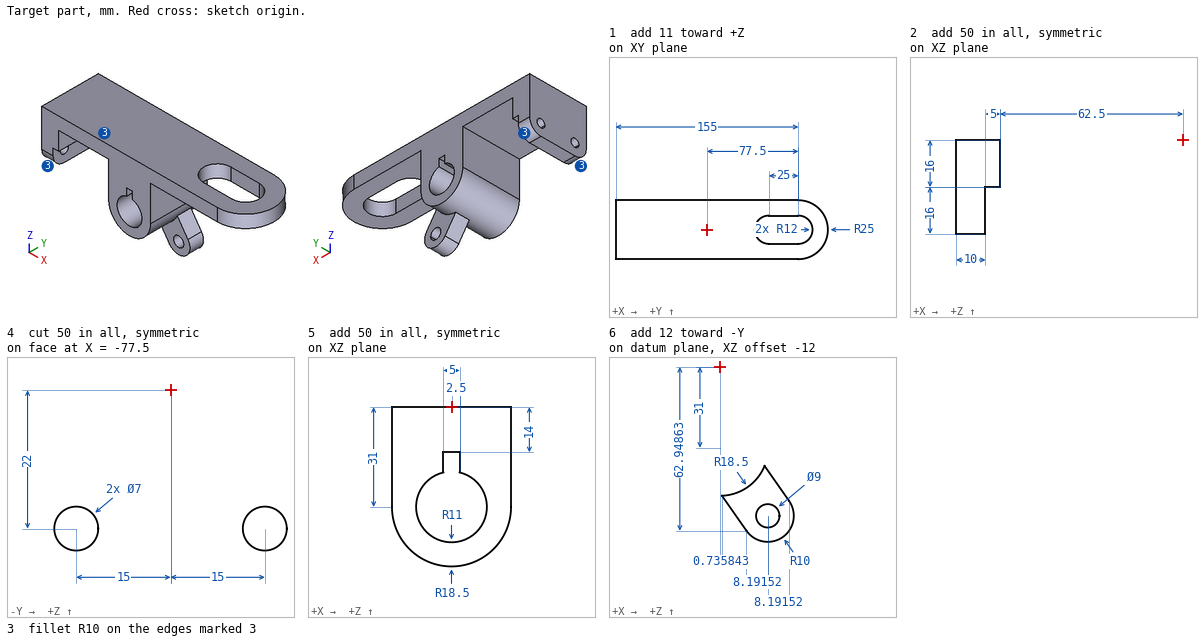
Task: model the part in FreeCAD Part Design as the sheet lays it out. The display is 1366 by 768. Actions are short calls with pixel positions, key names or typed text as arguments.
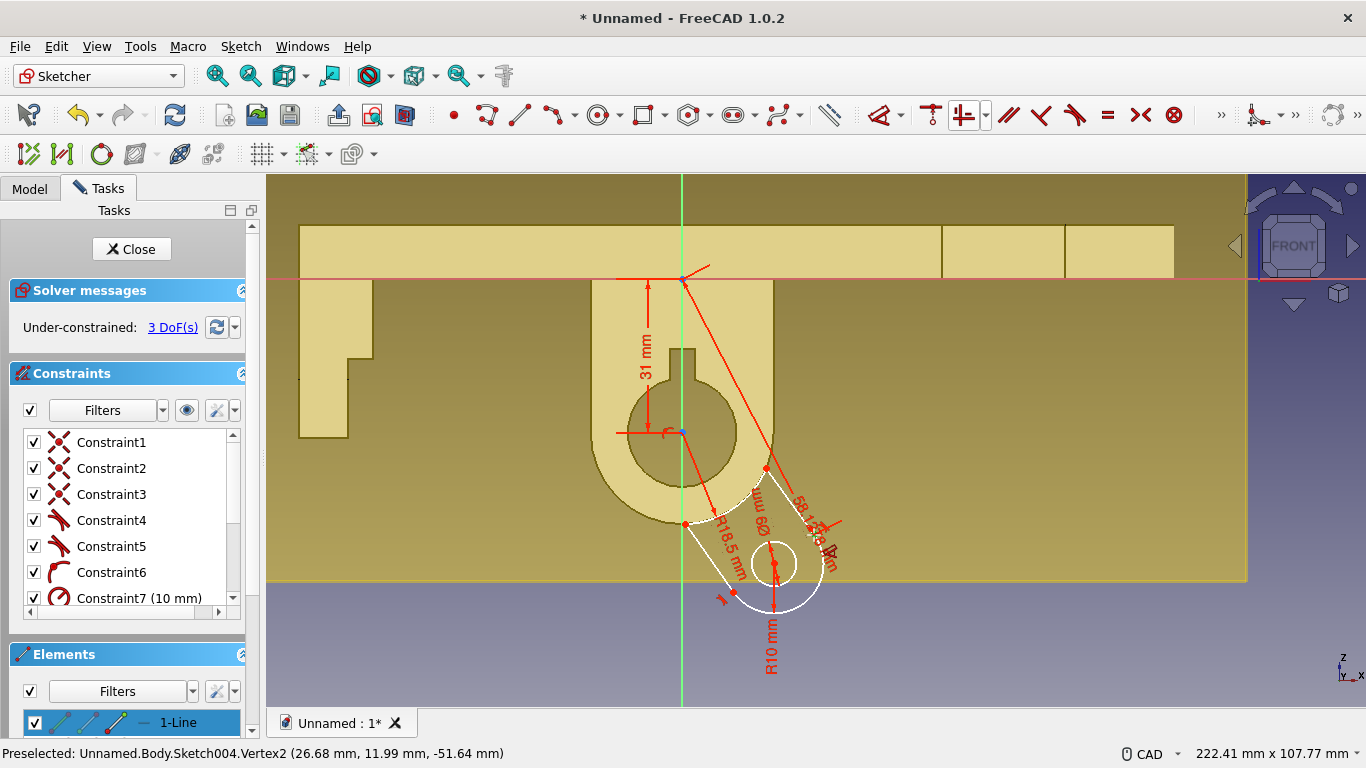
click(774, 564)
click(785, 598)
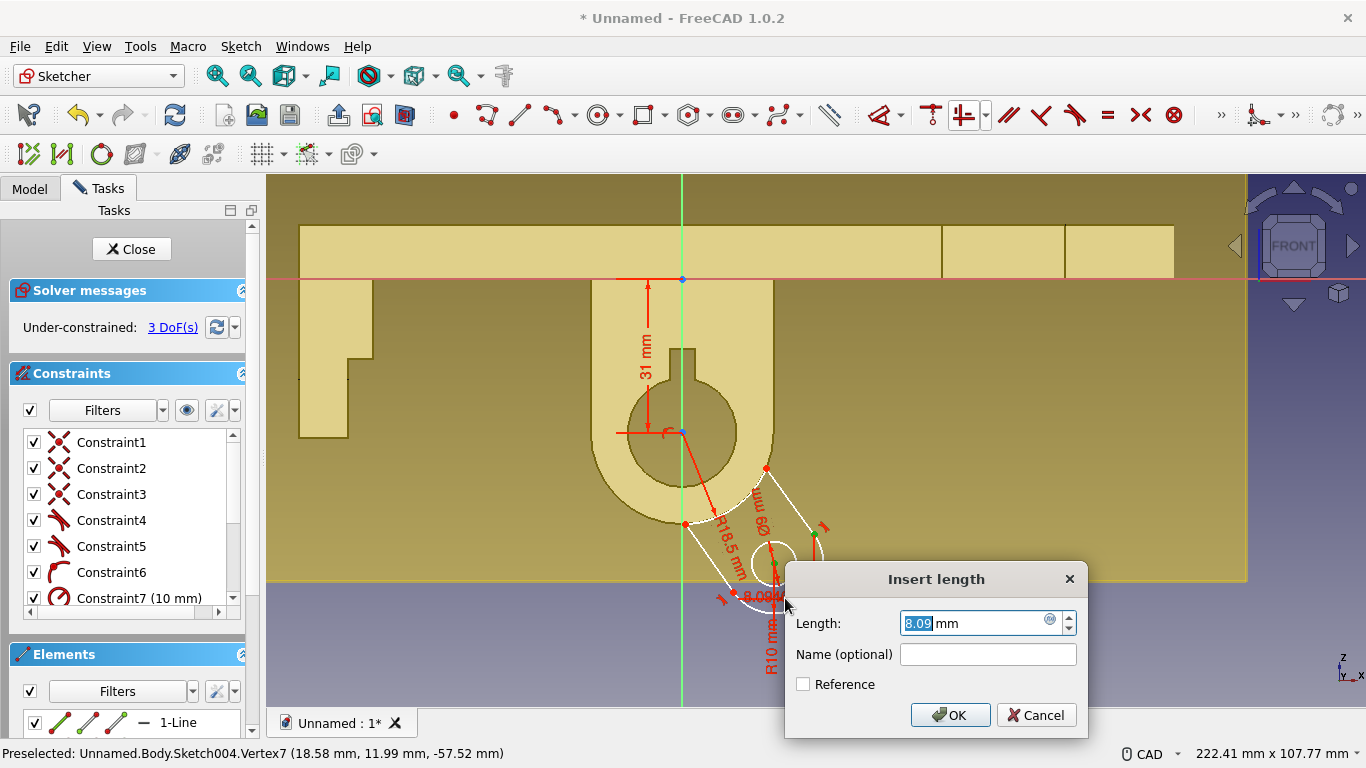
text(8.19152)
key(Return)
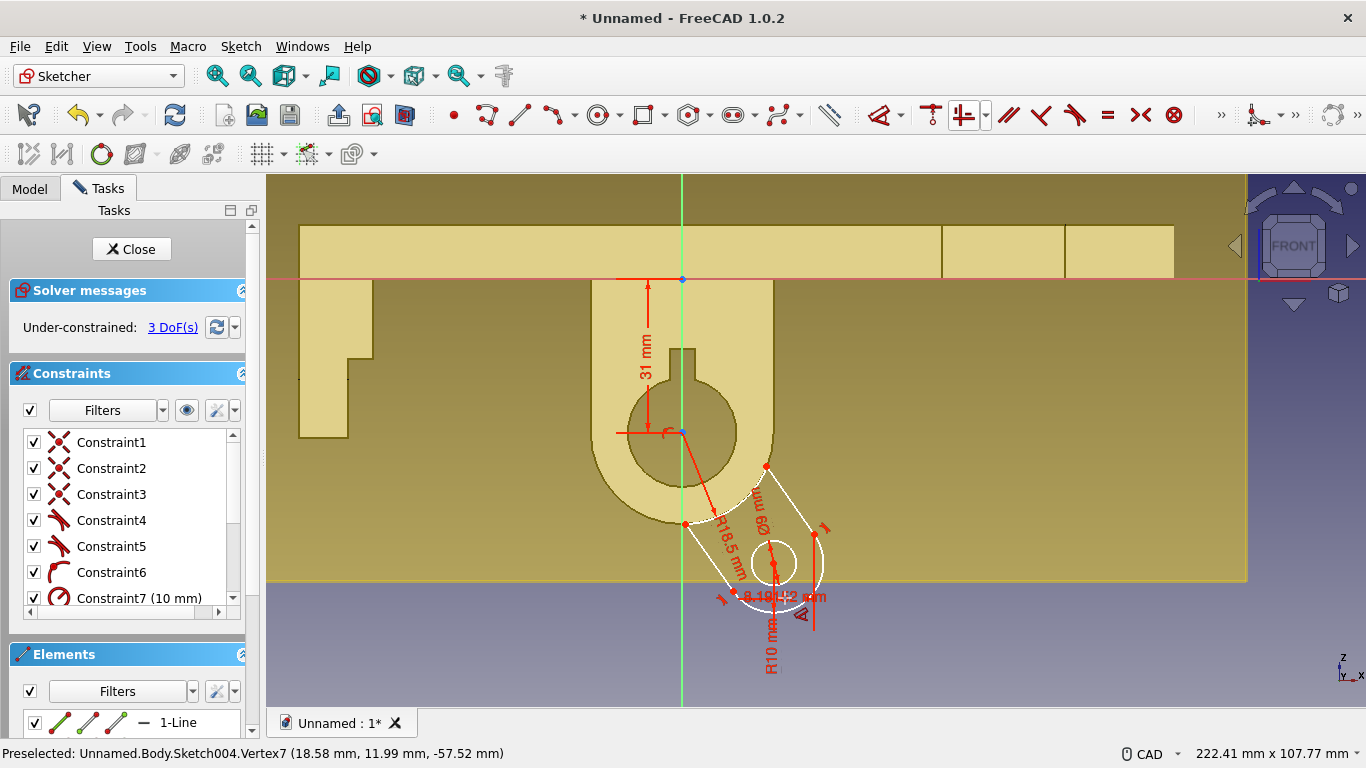
click(734, 592)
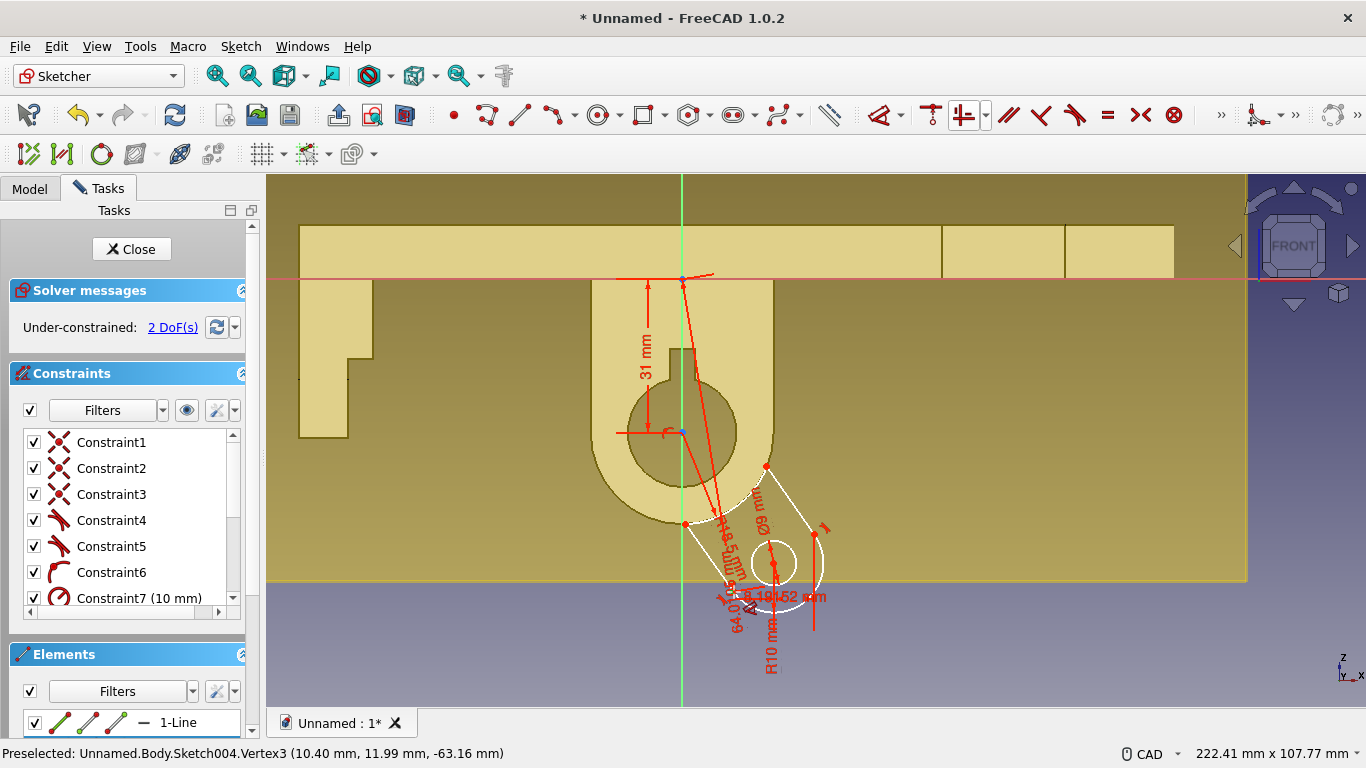
click(774, 563)
click(754, 626)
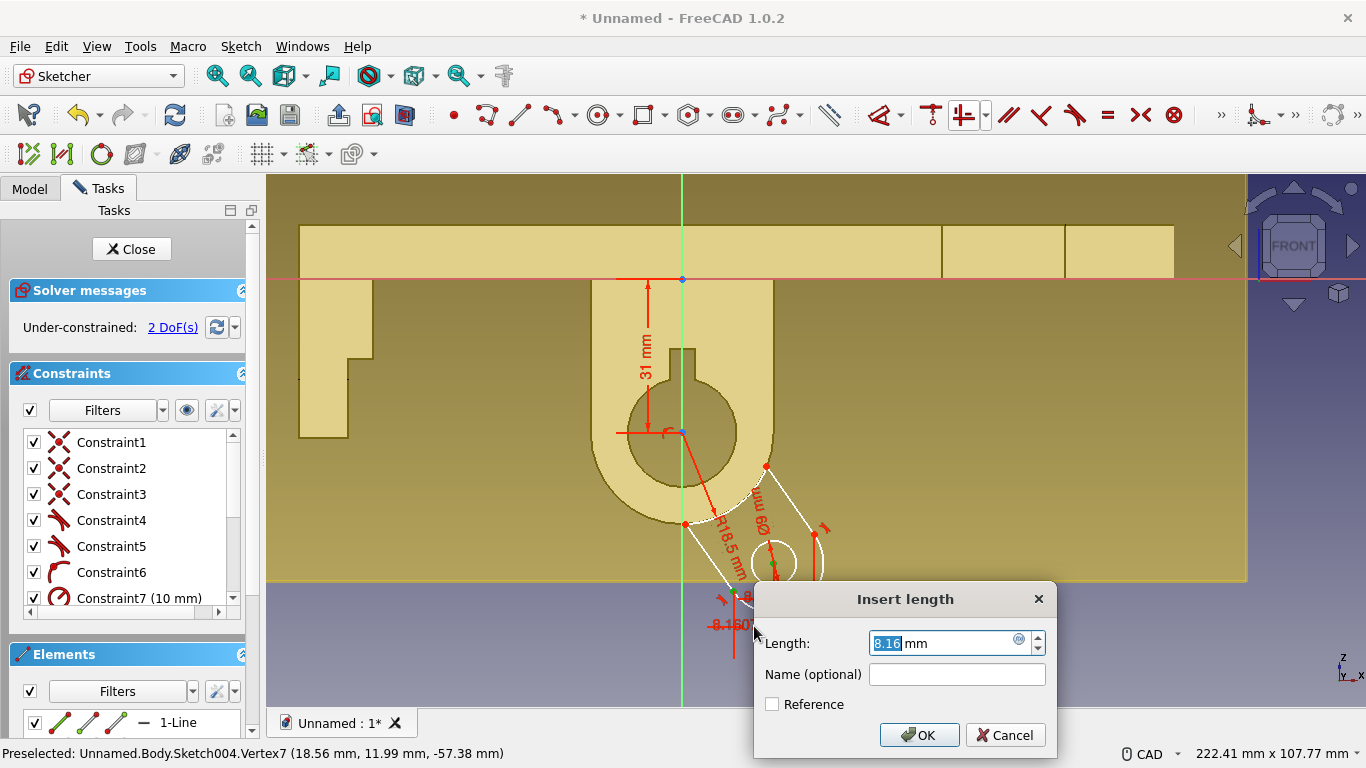
text(8.19152)
key(Return)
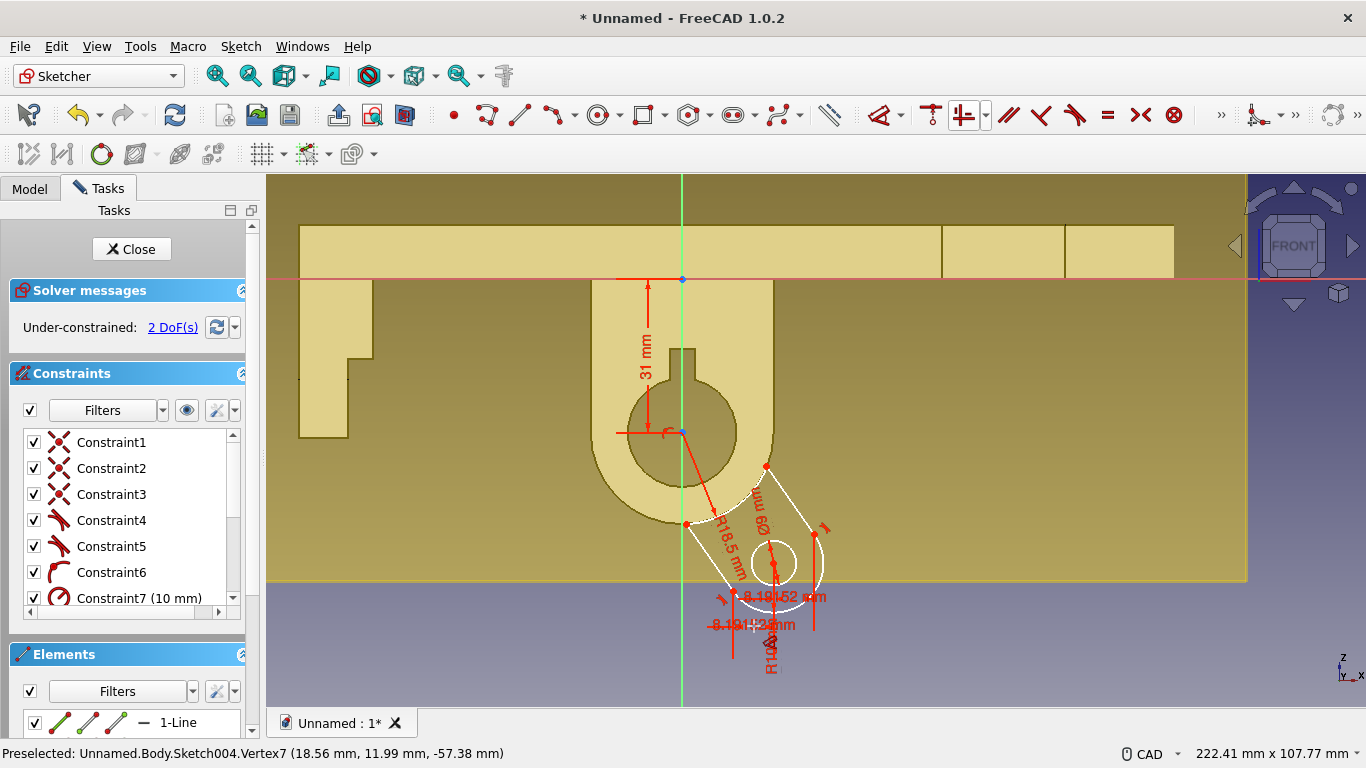
click(733, 592)
click(648, 435)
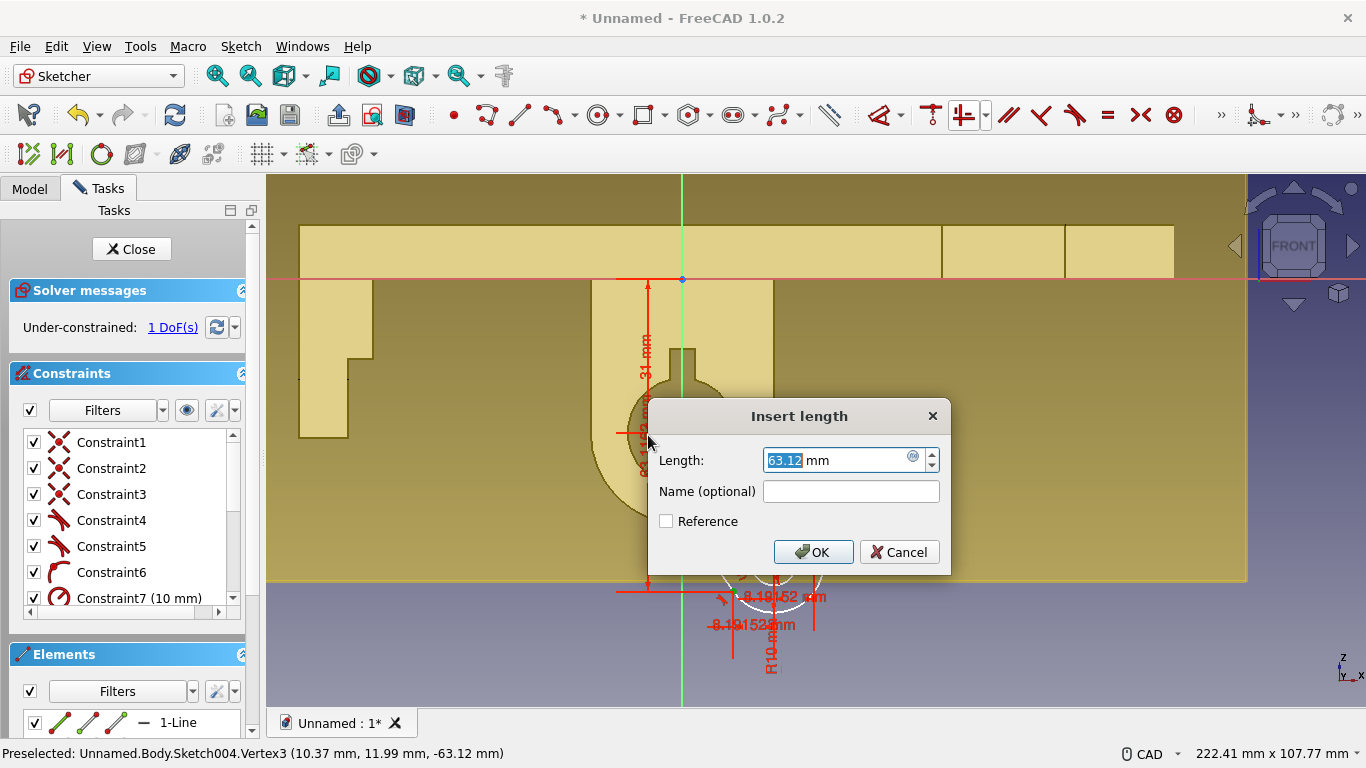
text(62.94863)
key(Return)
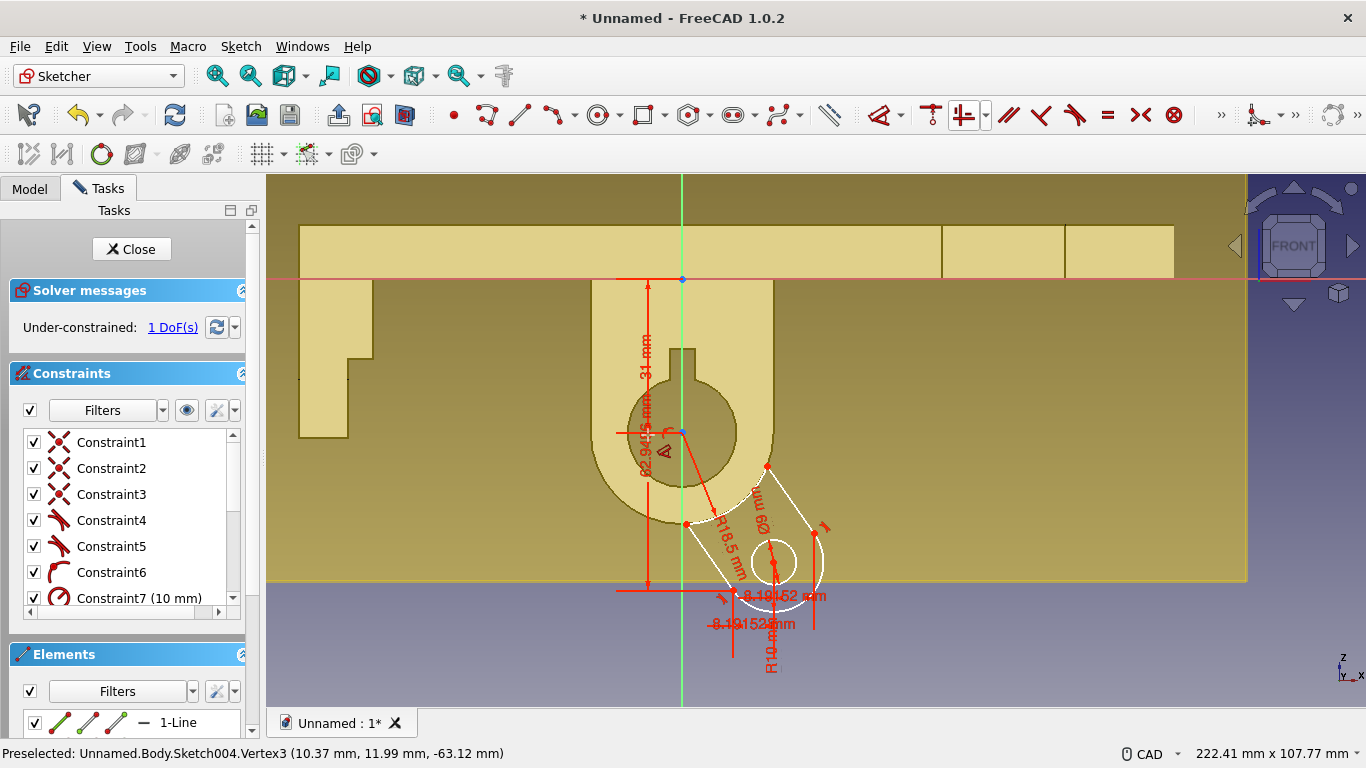
scroll(687, 524, up, 12)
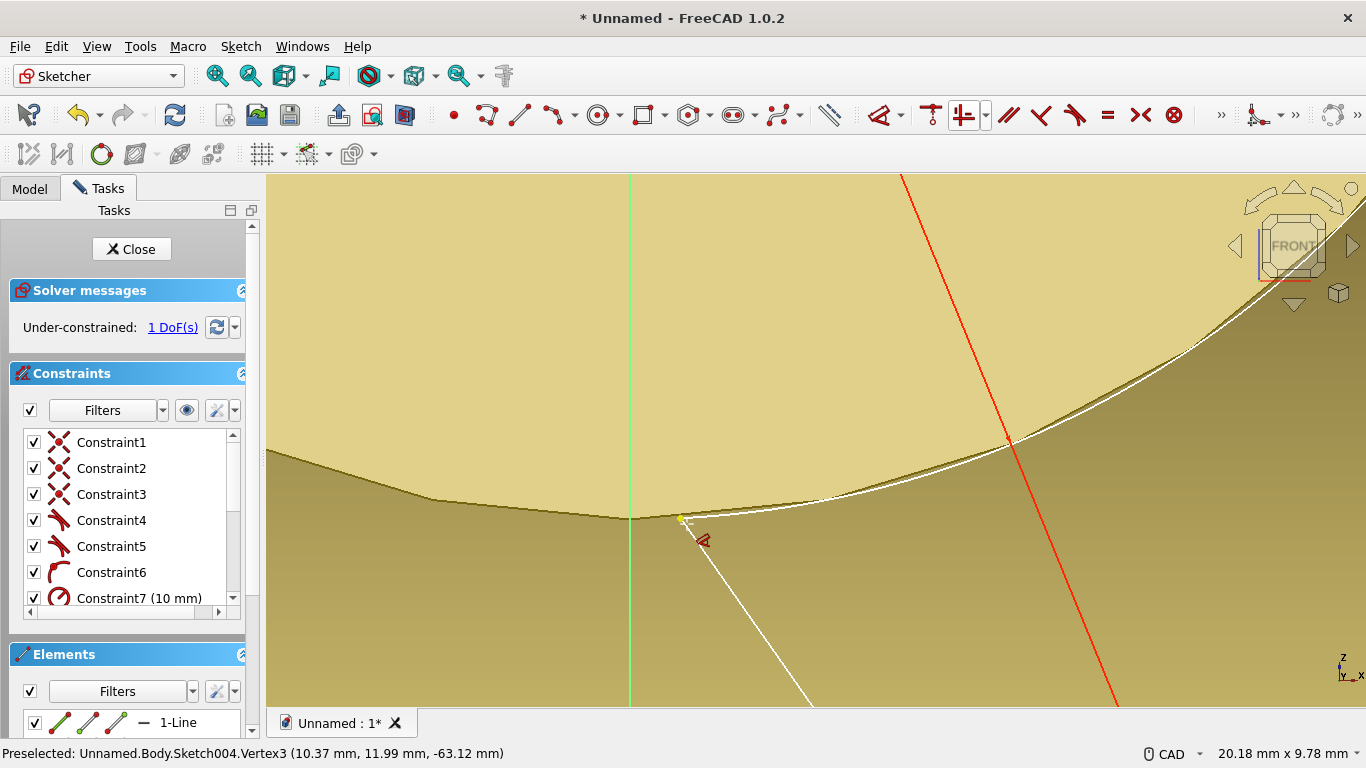
click(681, 518)
click(655, 552)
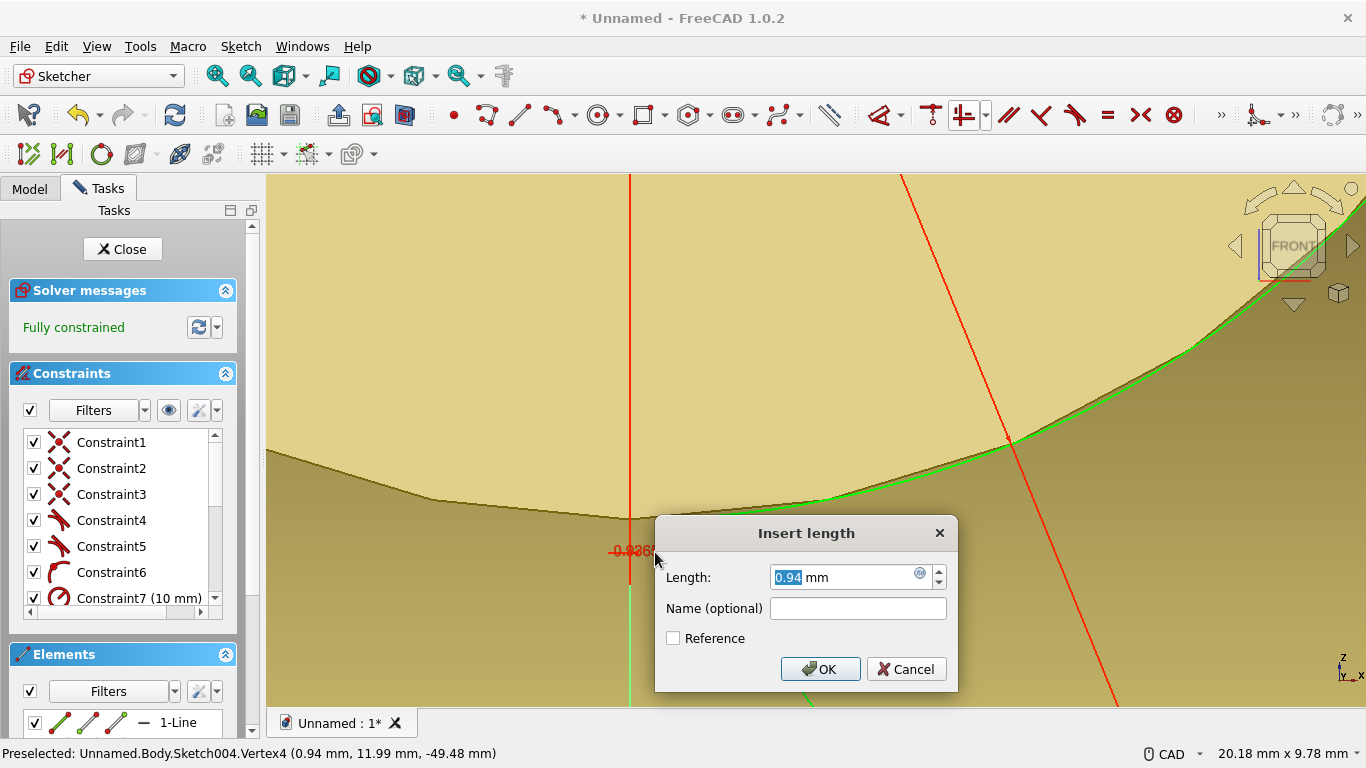
text(0.735843)
key(Return)
key(Escape)